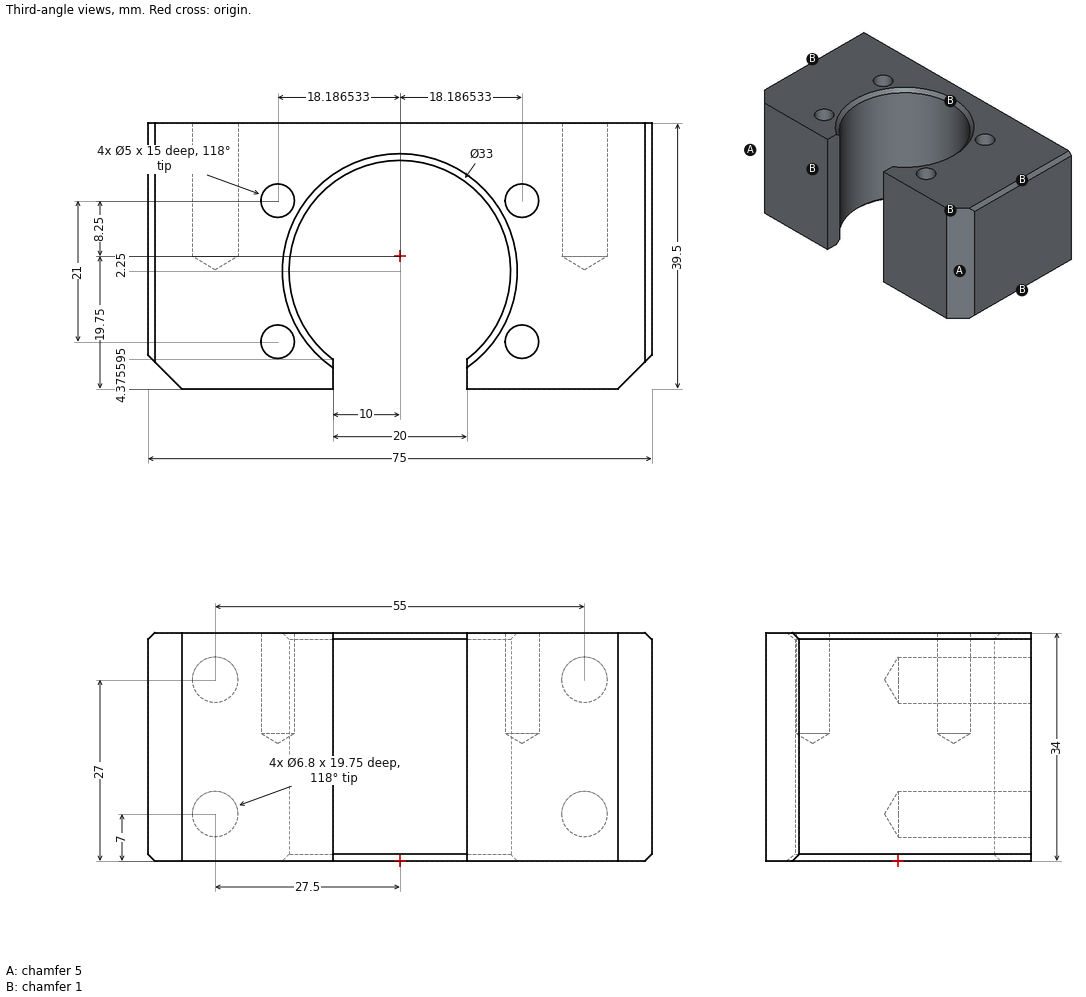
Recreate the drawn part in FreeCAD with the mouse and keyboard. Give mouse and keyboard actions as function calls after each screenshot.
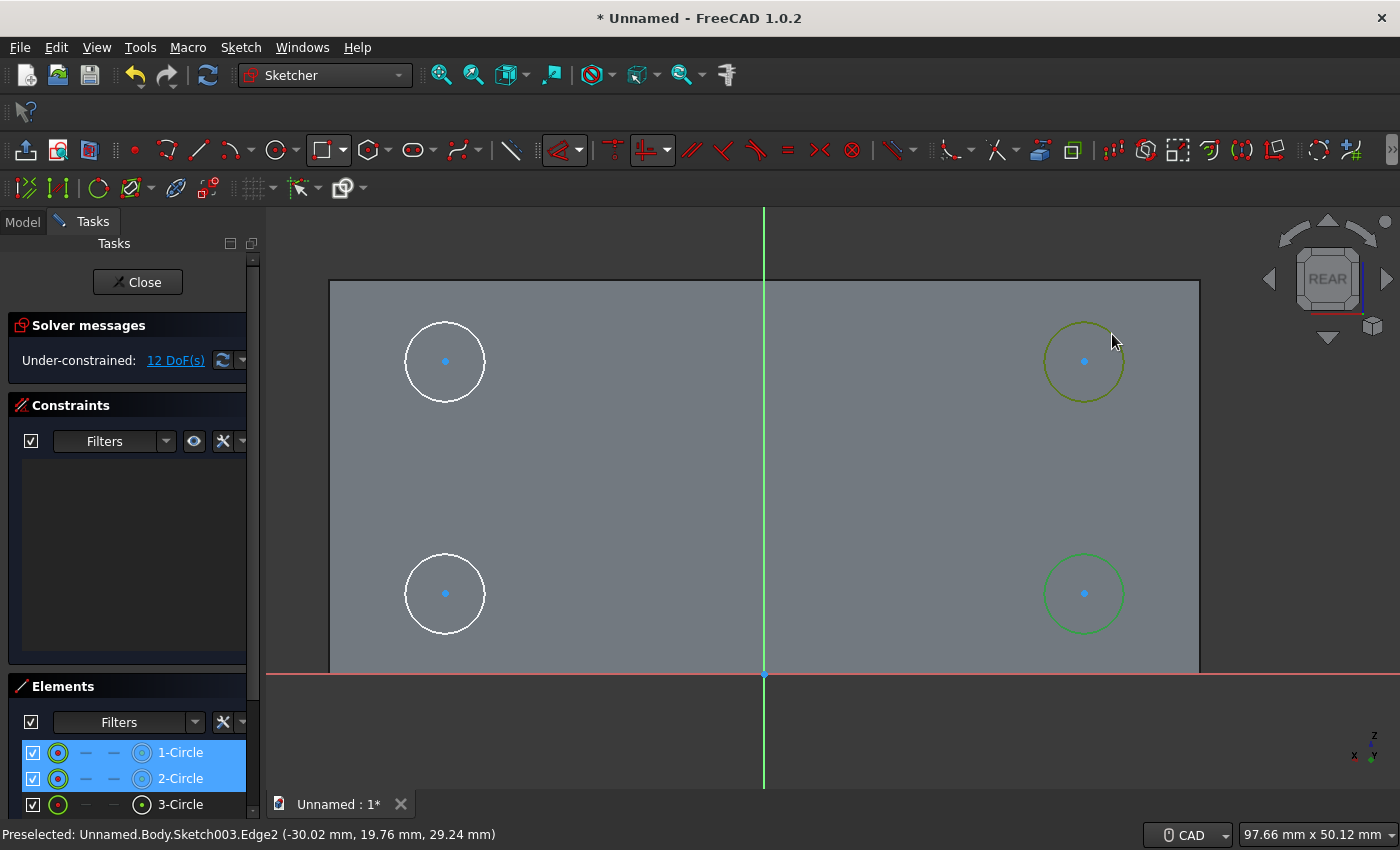
click(473, 334)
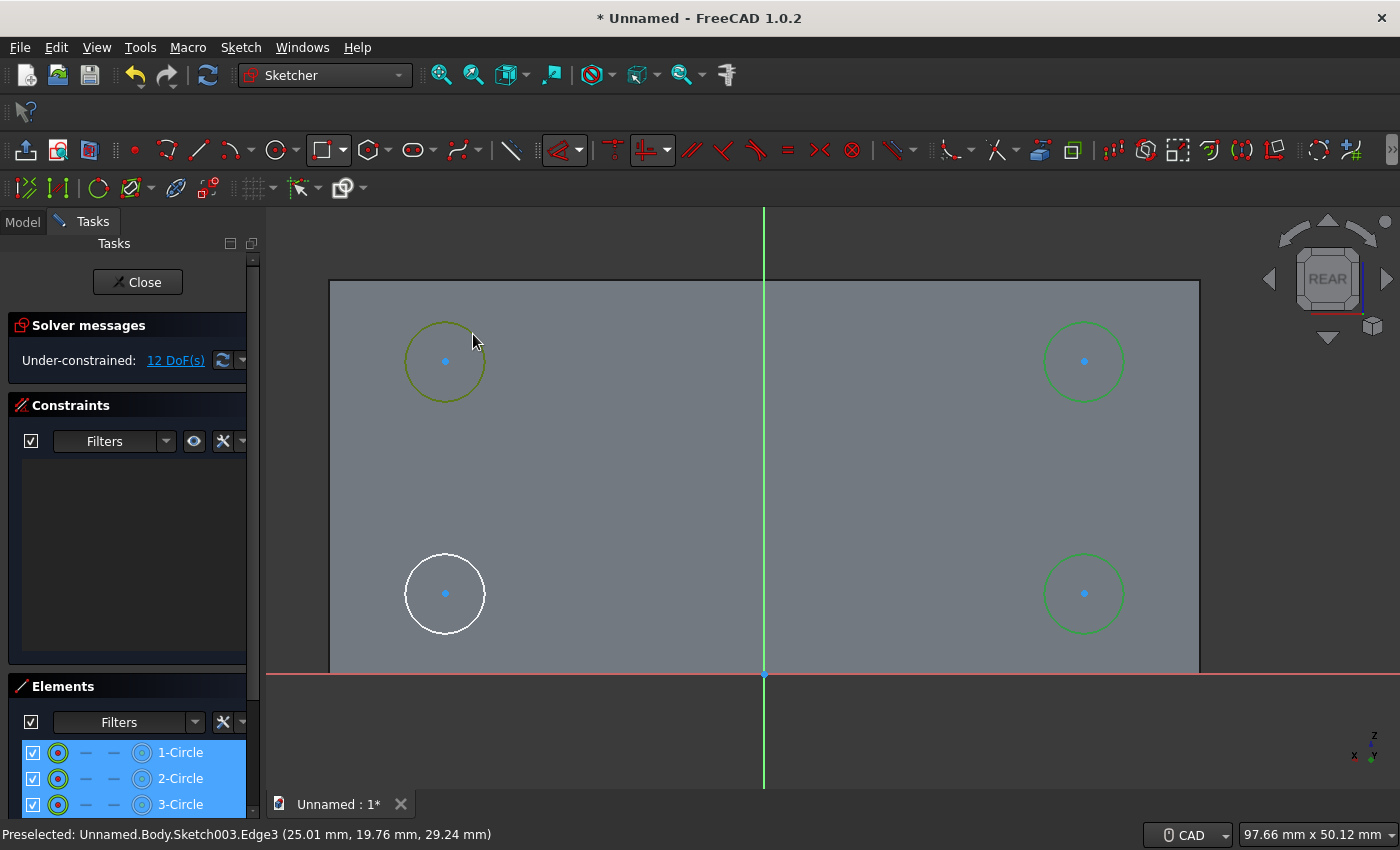
click(473, 566)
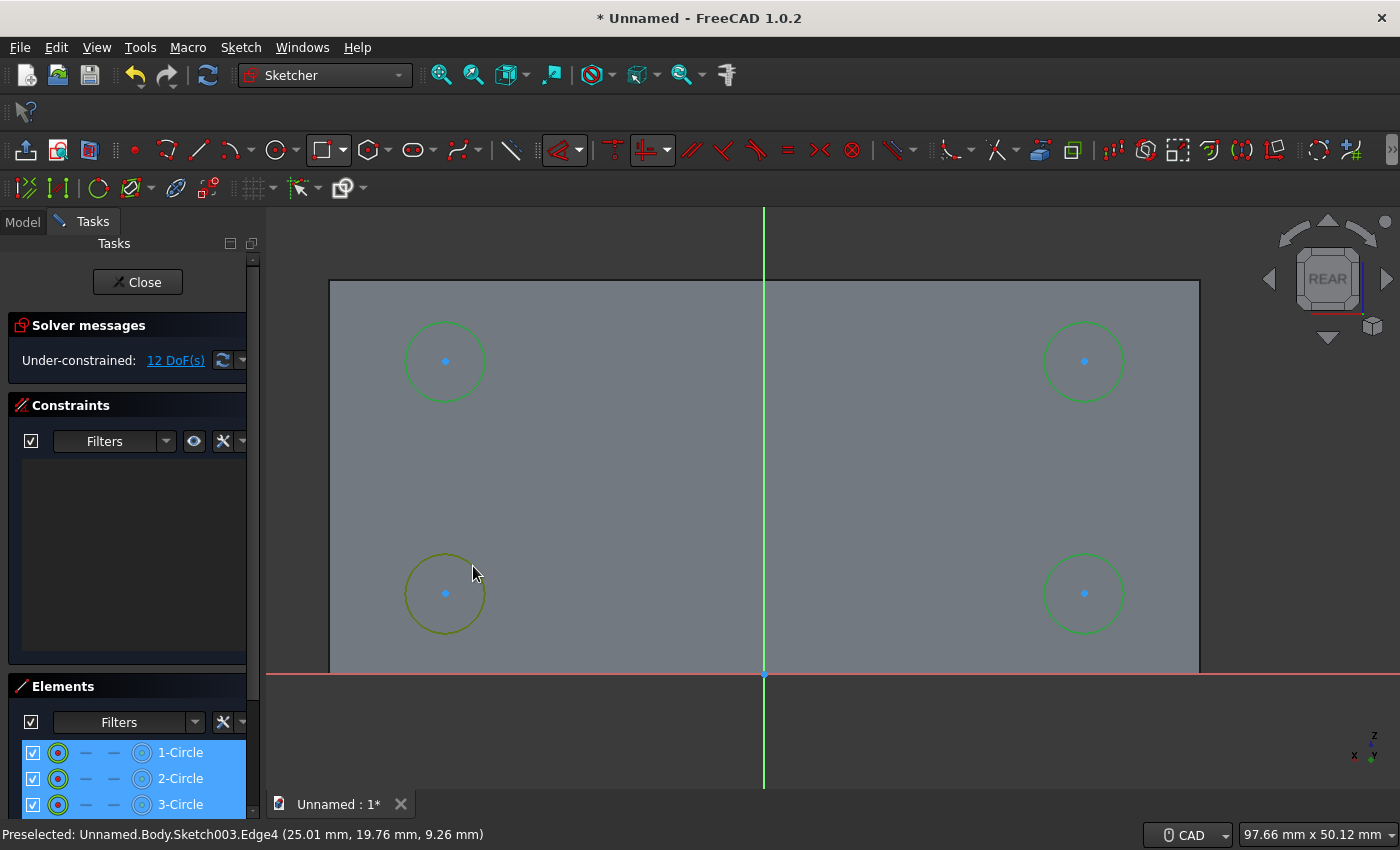
click(788, 150)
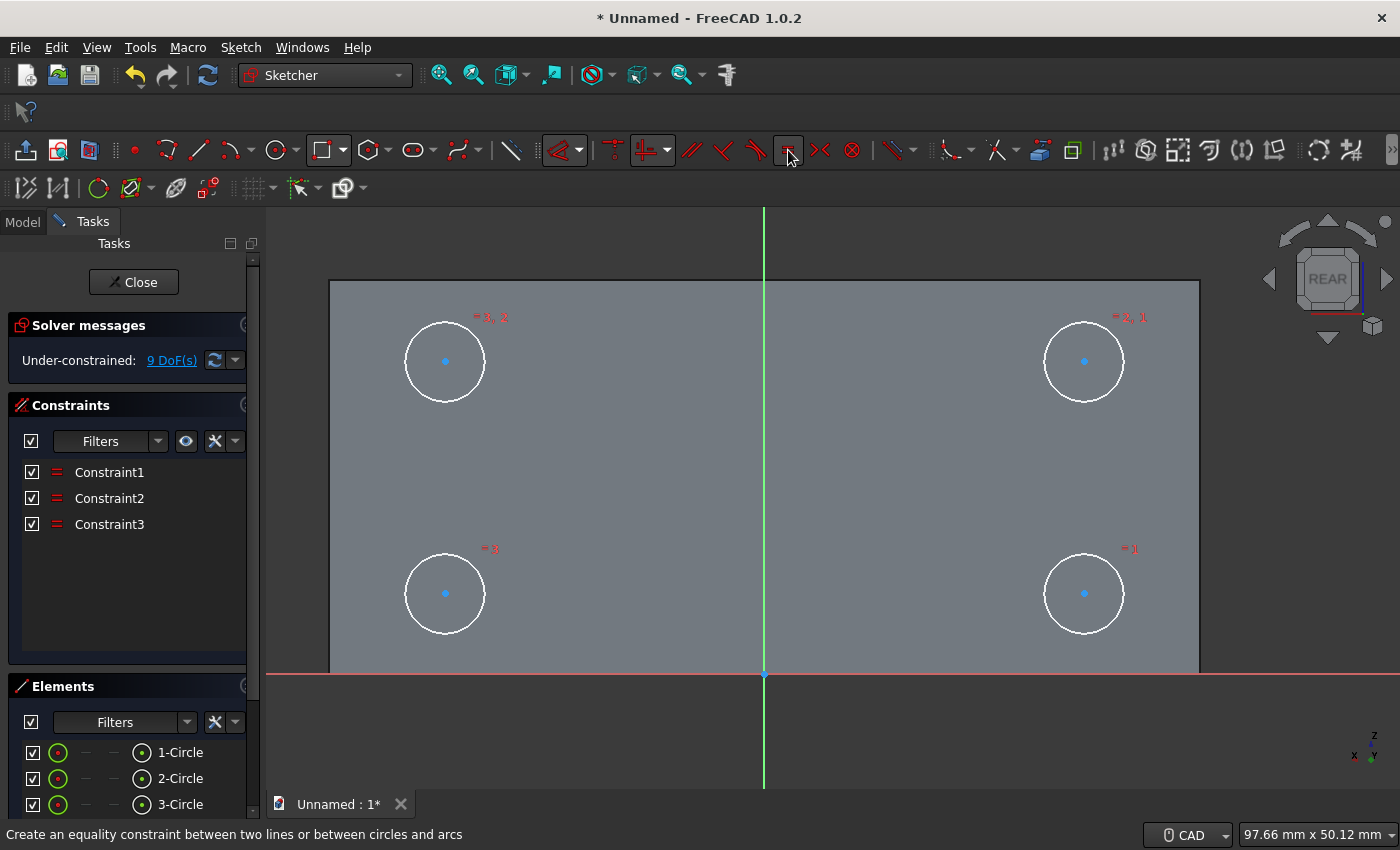
click(1084, 594)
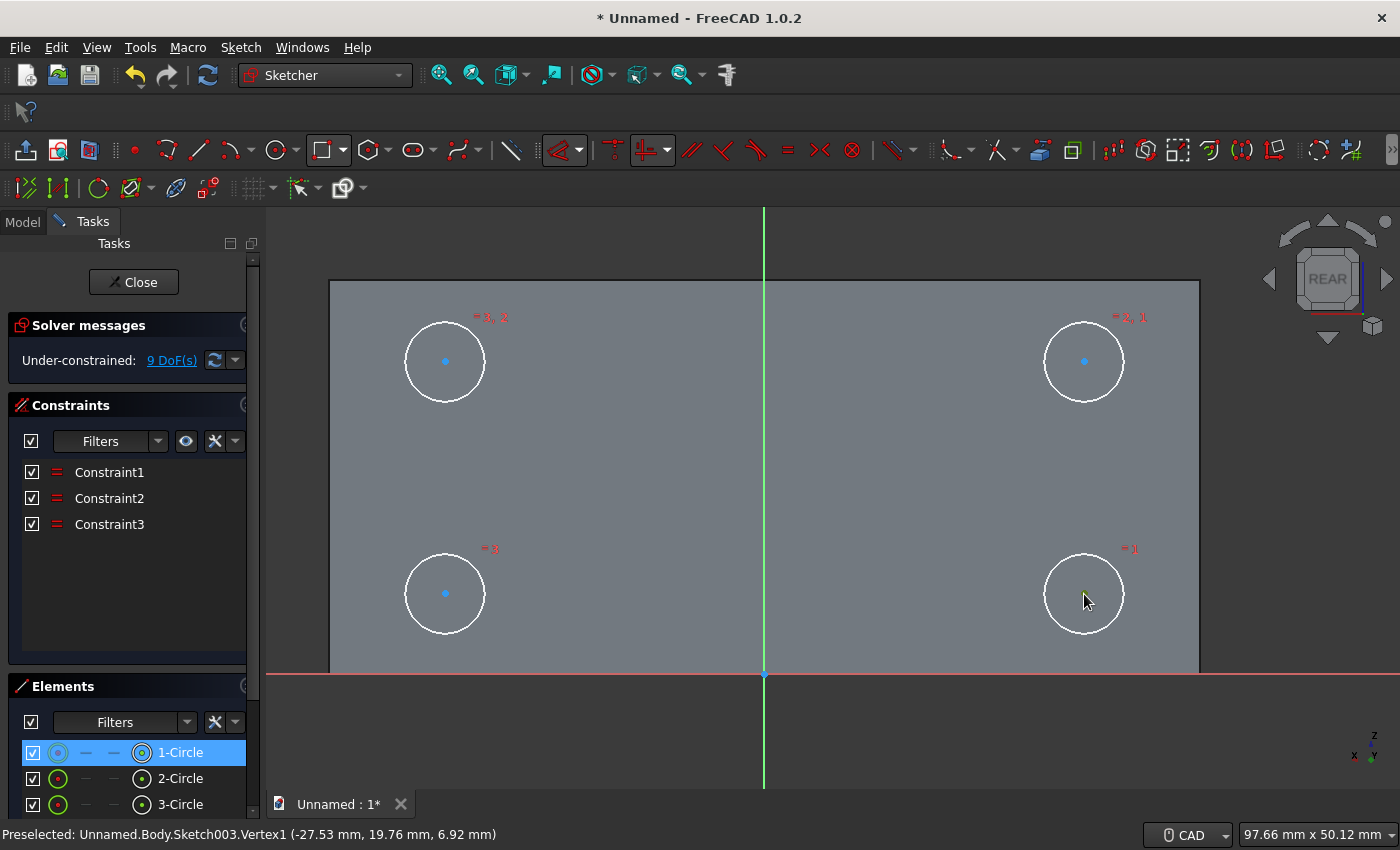
click(1084, 362)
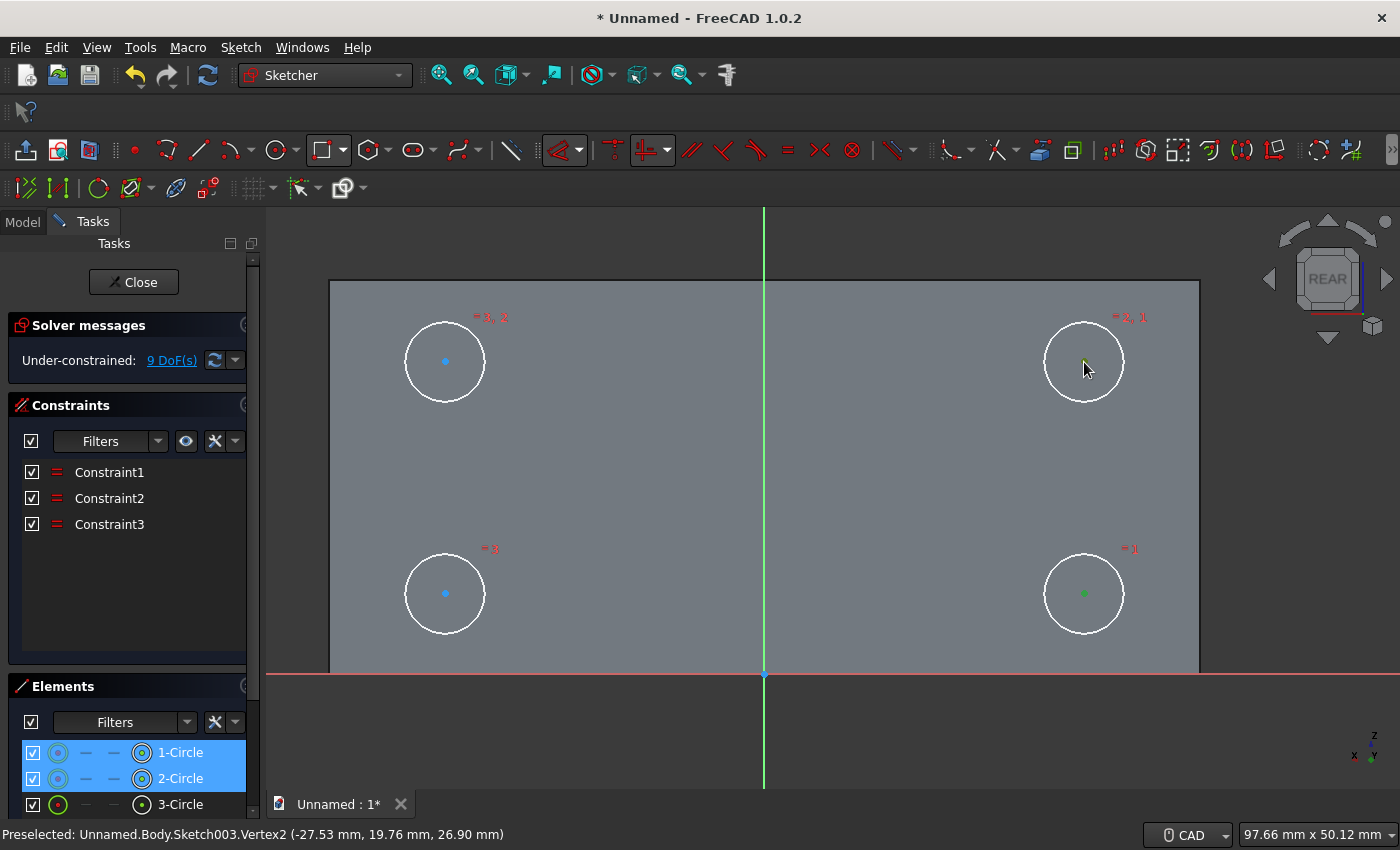
key(v)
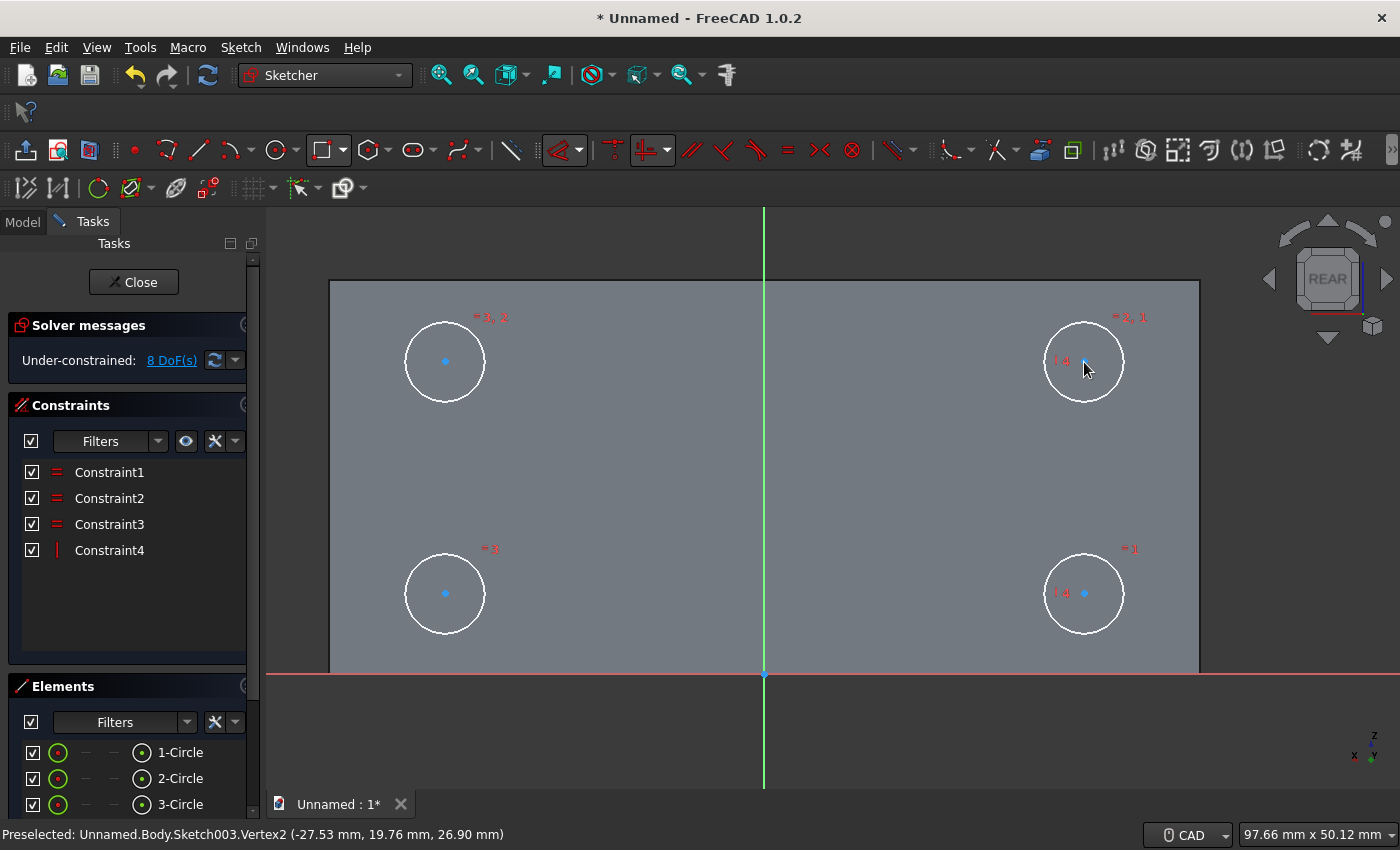
click(1084, 362)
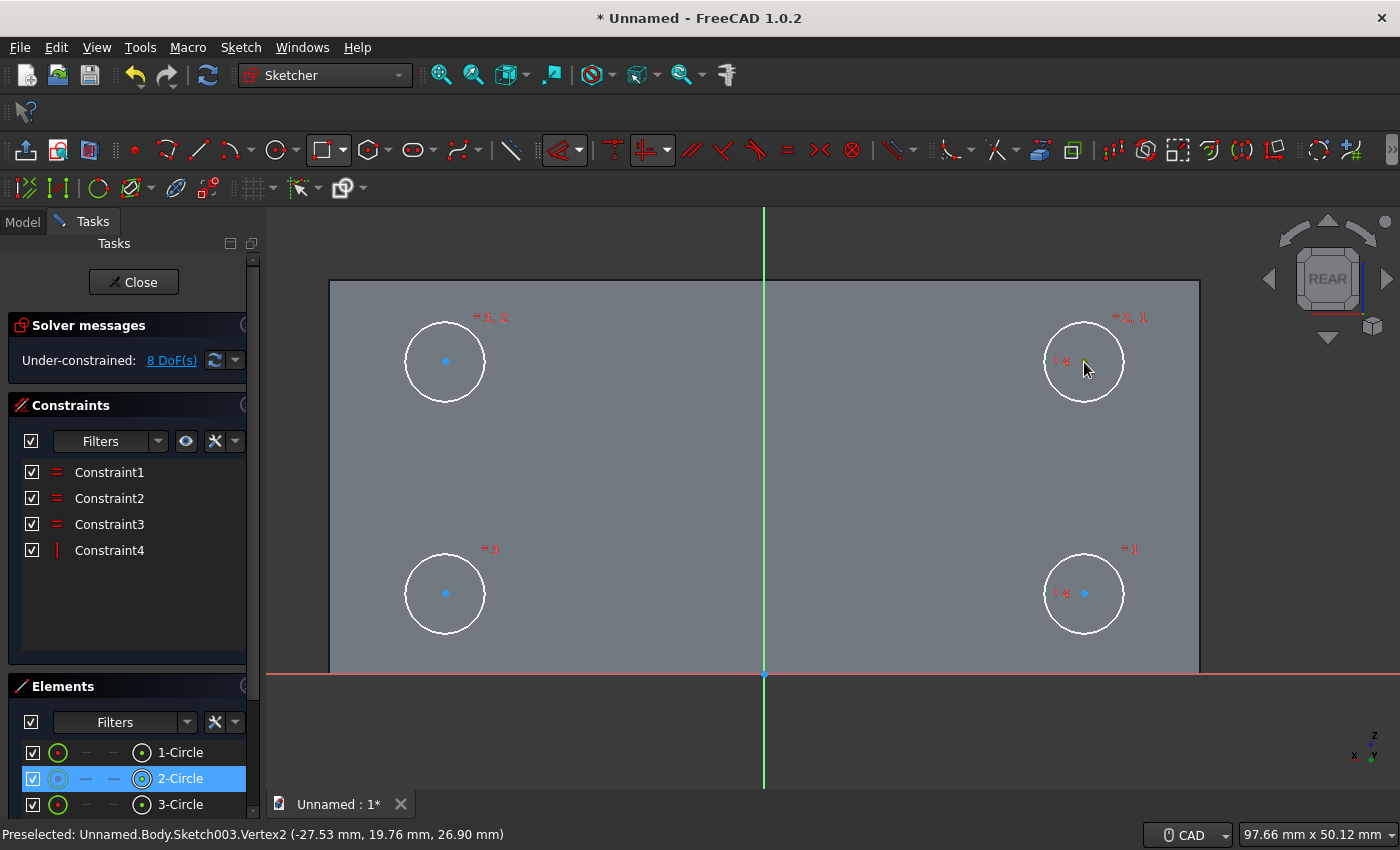
click(445, 362)